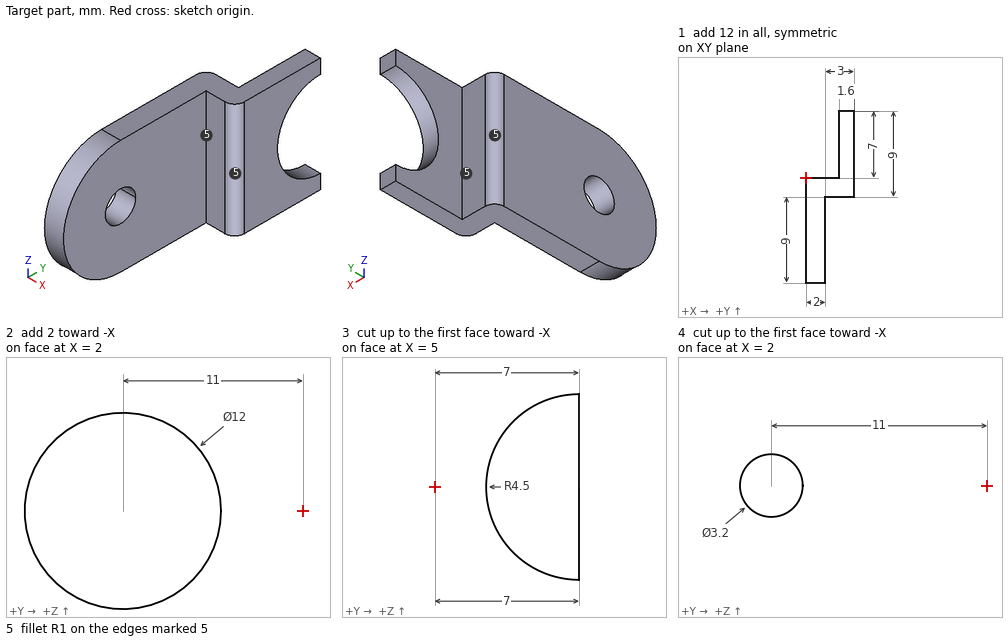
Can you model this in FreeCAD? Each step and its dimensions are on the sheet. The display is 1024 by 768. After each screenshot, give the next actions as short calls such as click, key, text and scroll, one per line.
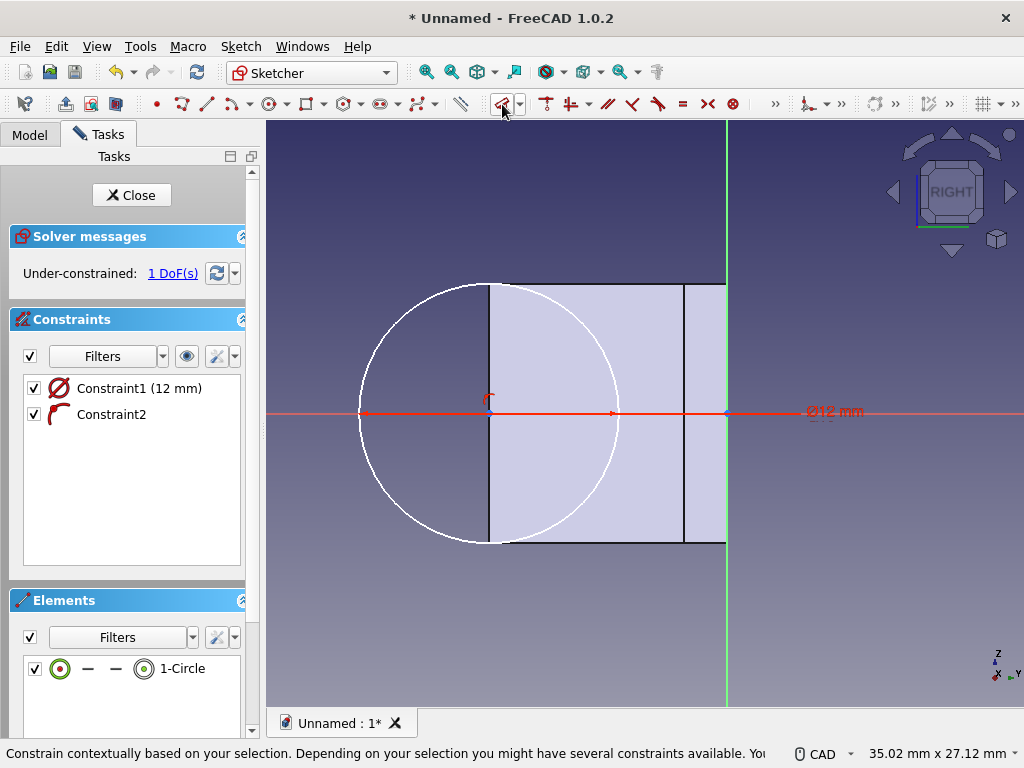
click(489, 414)
click(553, 448)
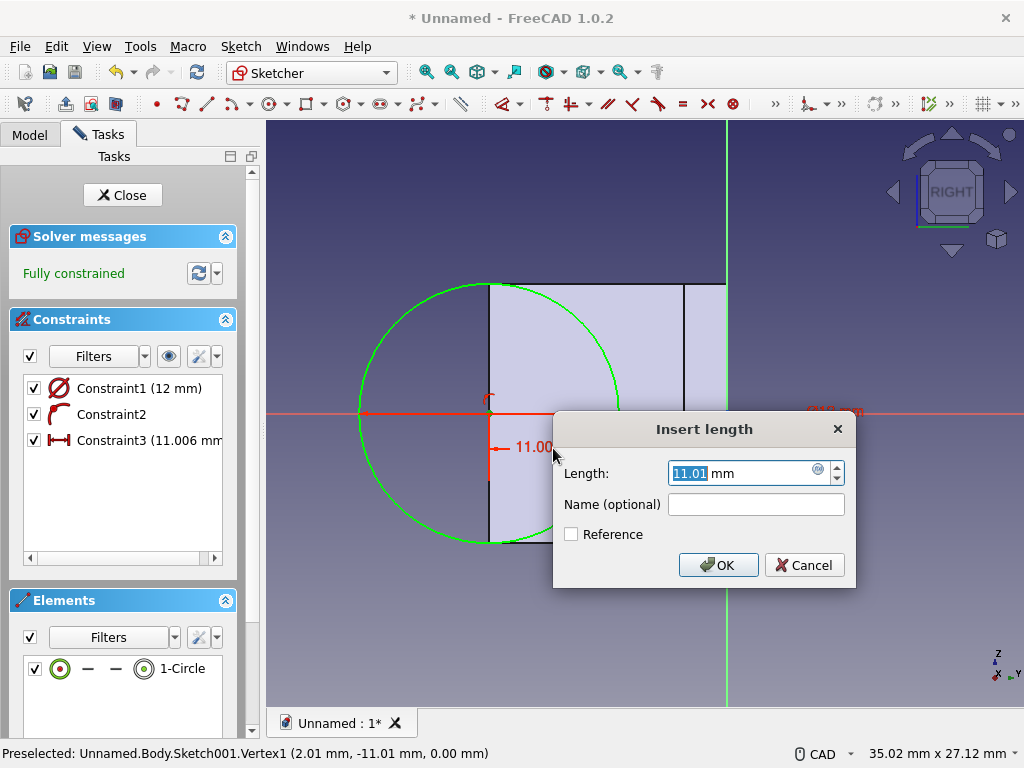
text(11)
key(Return)
key(Escape)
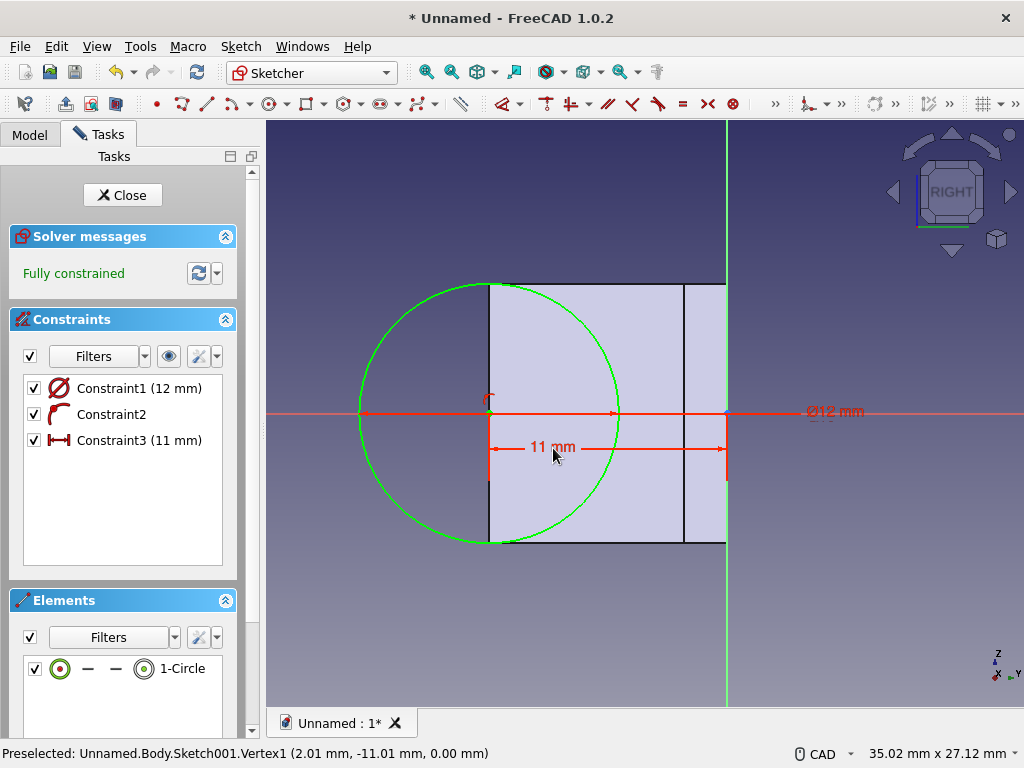
click(123, 195)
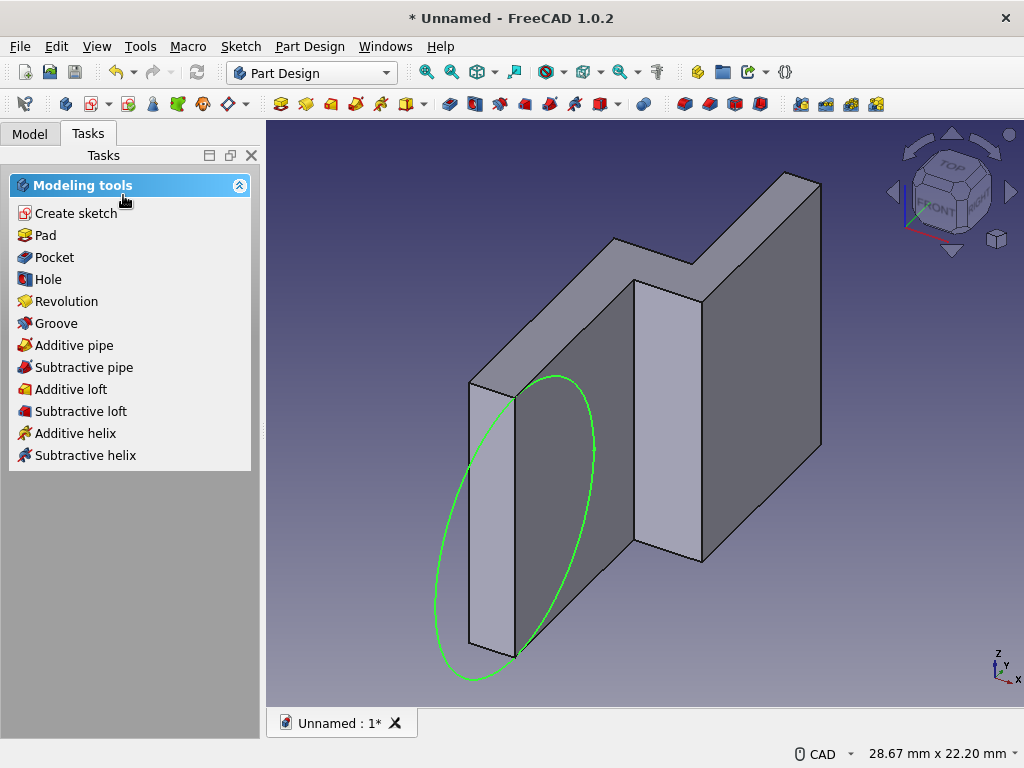
click(281, 104)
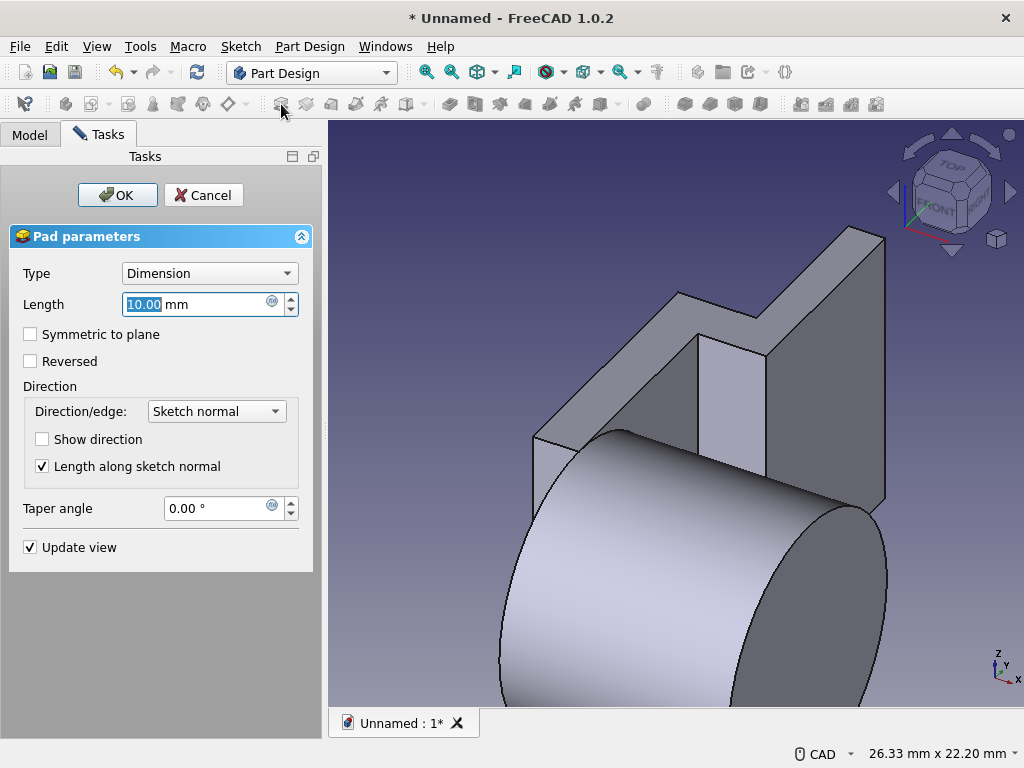
text(2)
key(Tab)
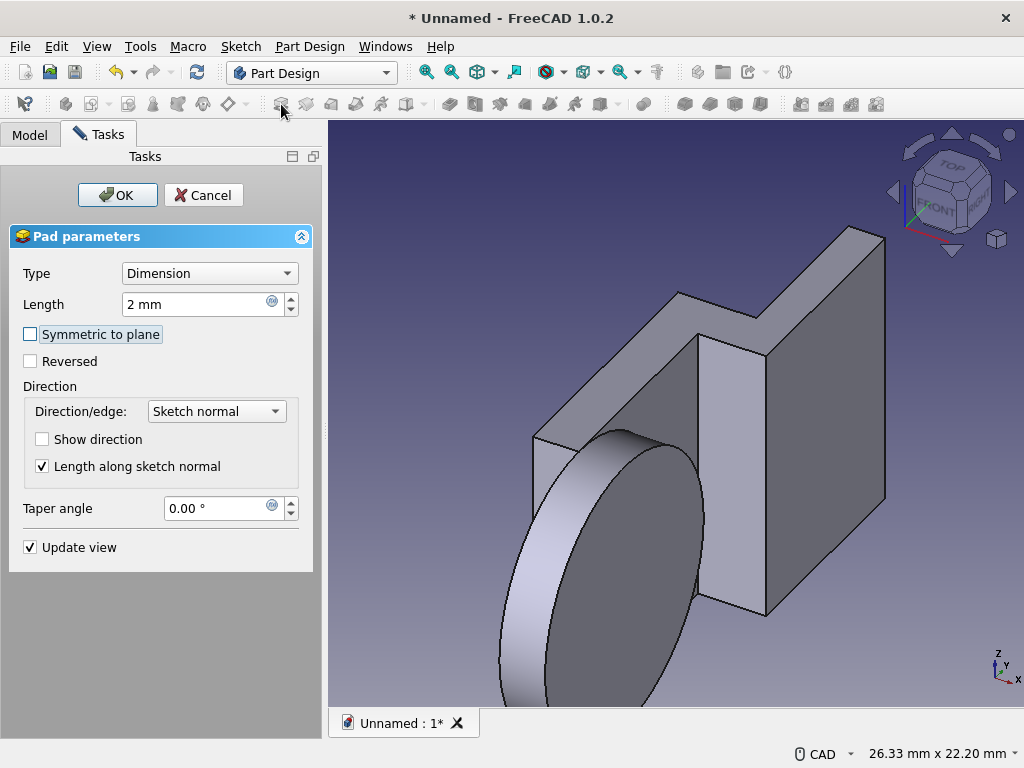
click(31, 361)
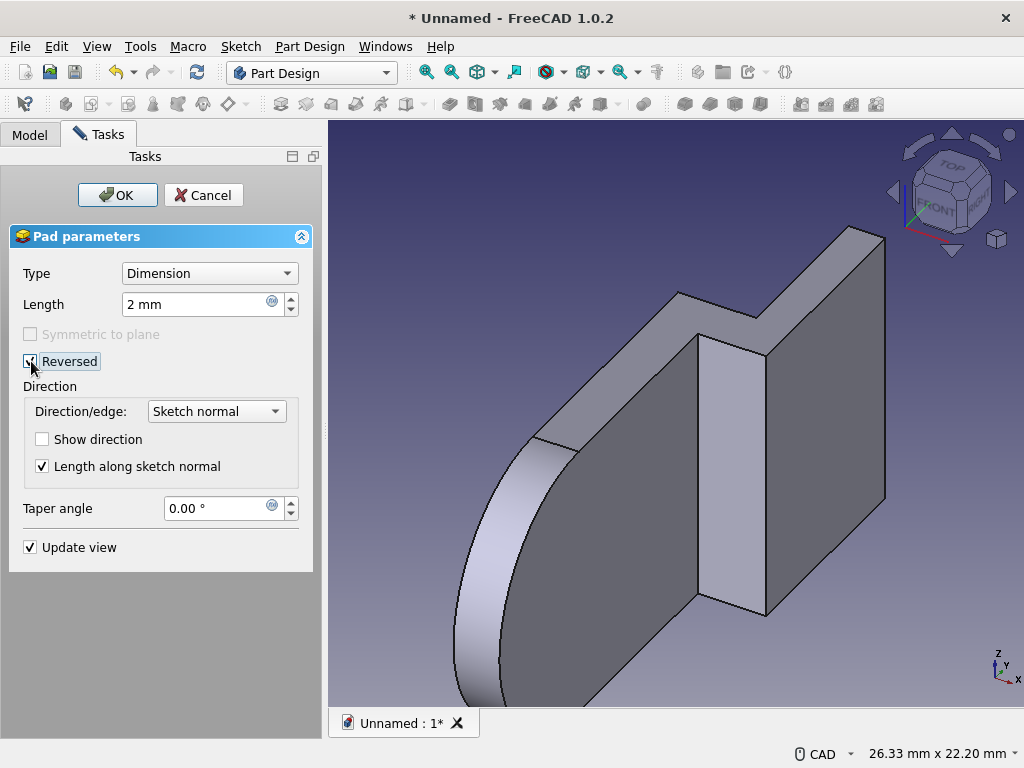
click(118, 195)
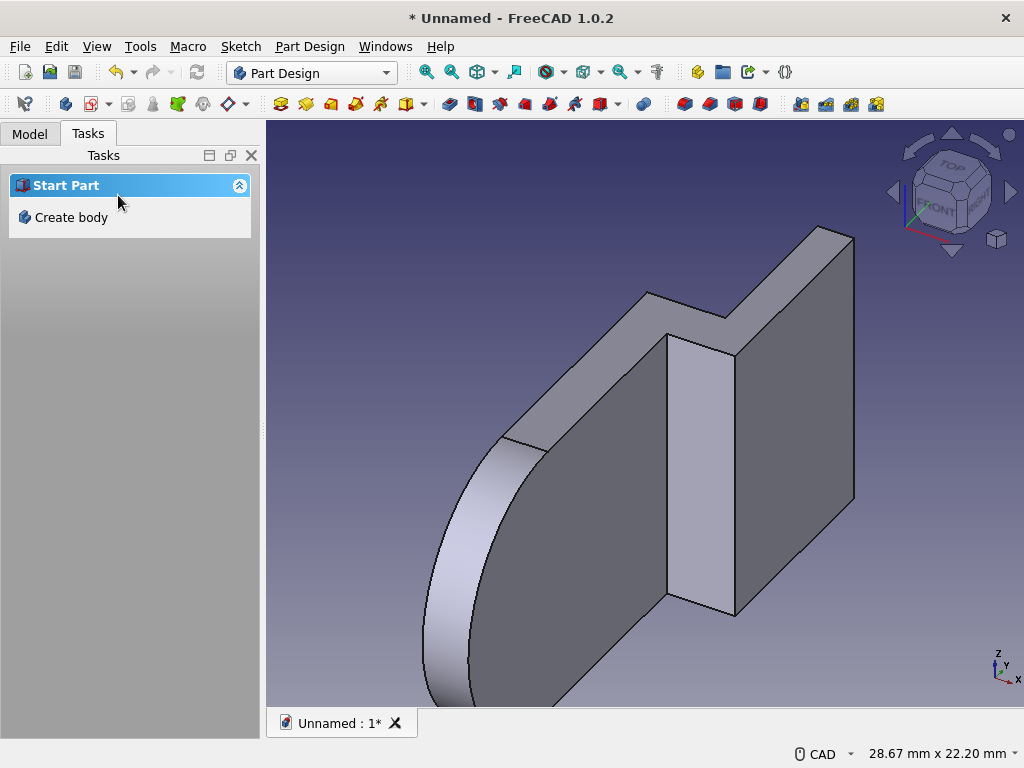
key(v)
key(f)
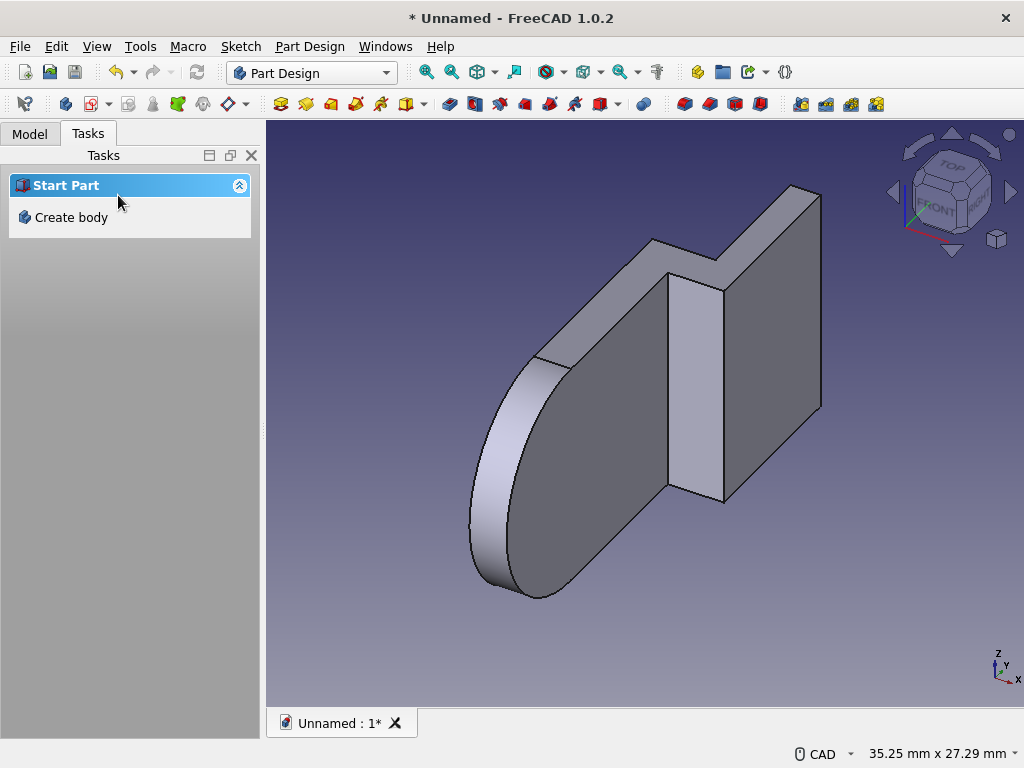
click(772, 348)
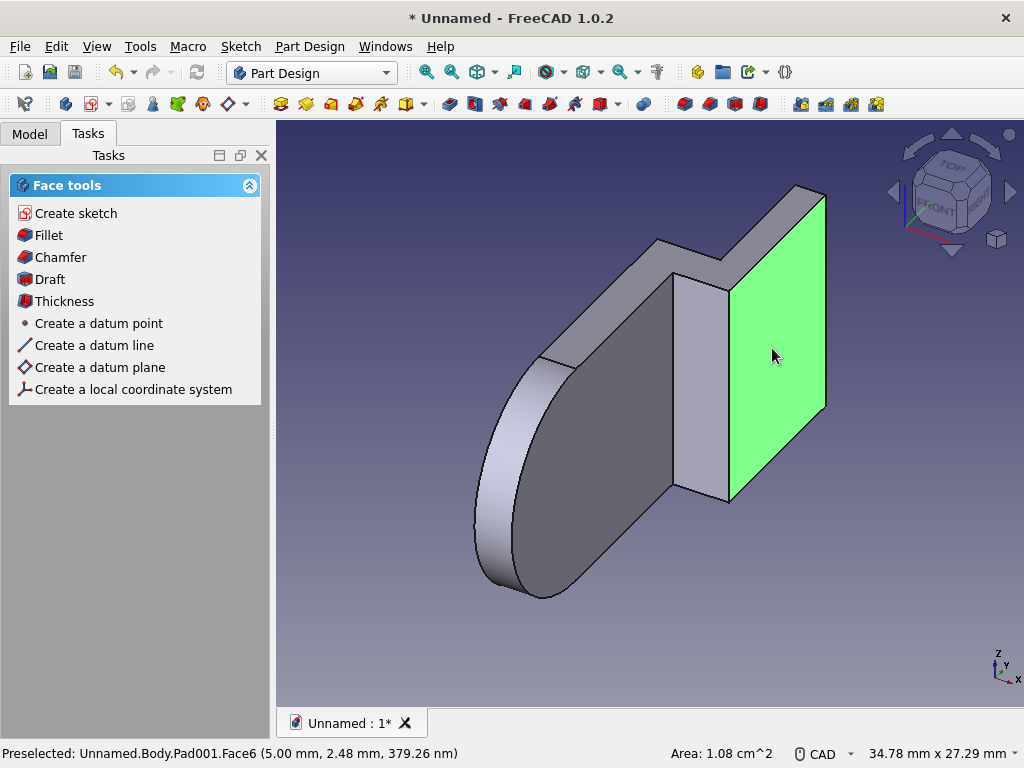
click(90, 104)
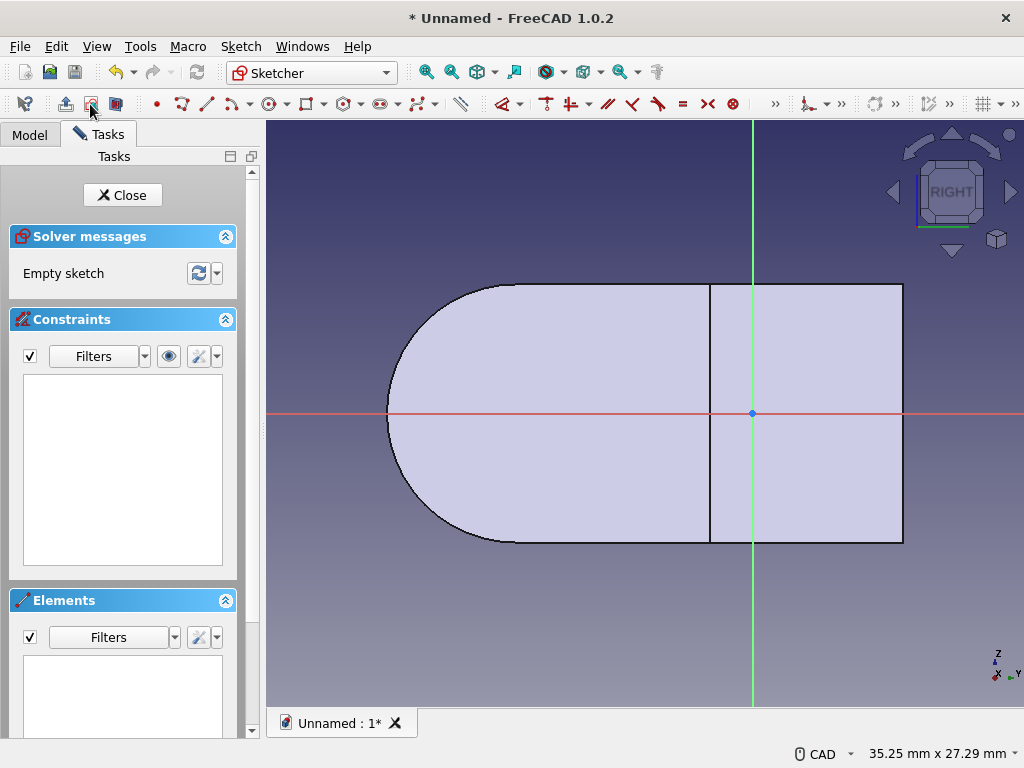
scroll(576, 414, down, 5)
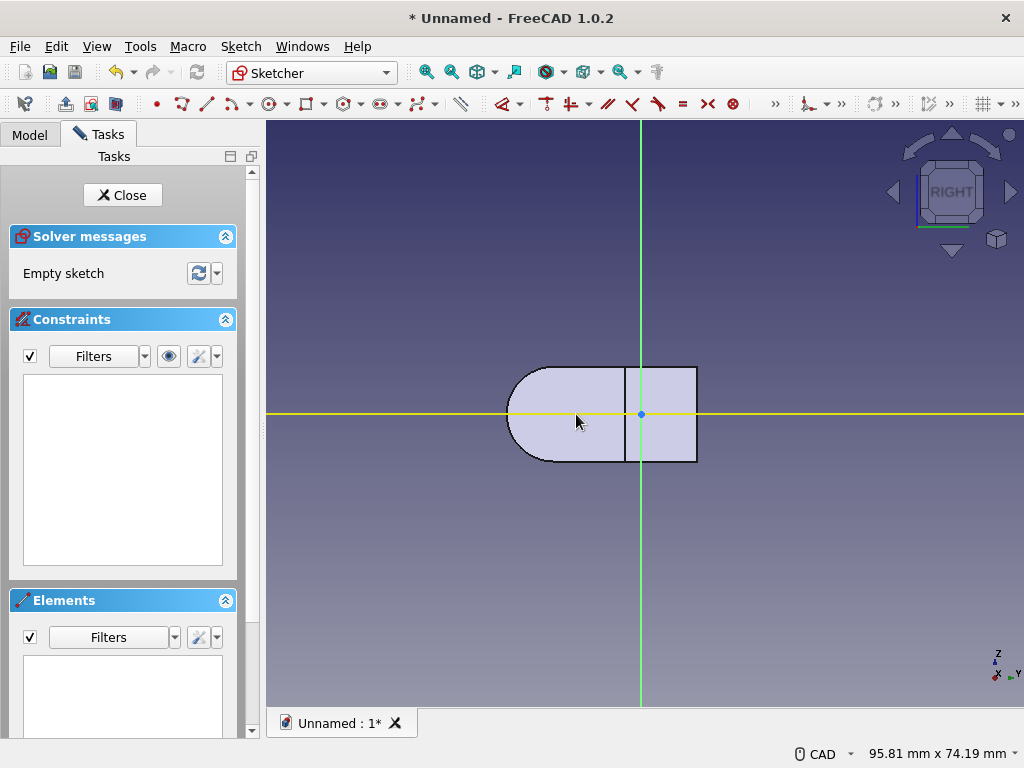
scroll(692, 414, up, 8)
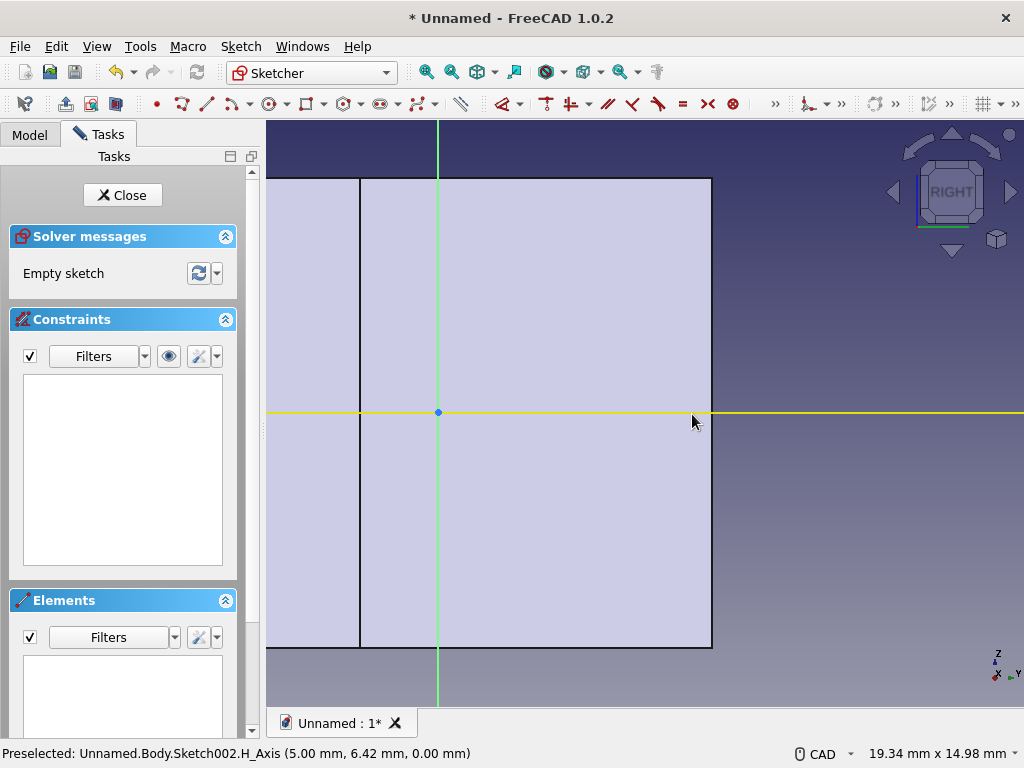
key(g)
key(l)